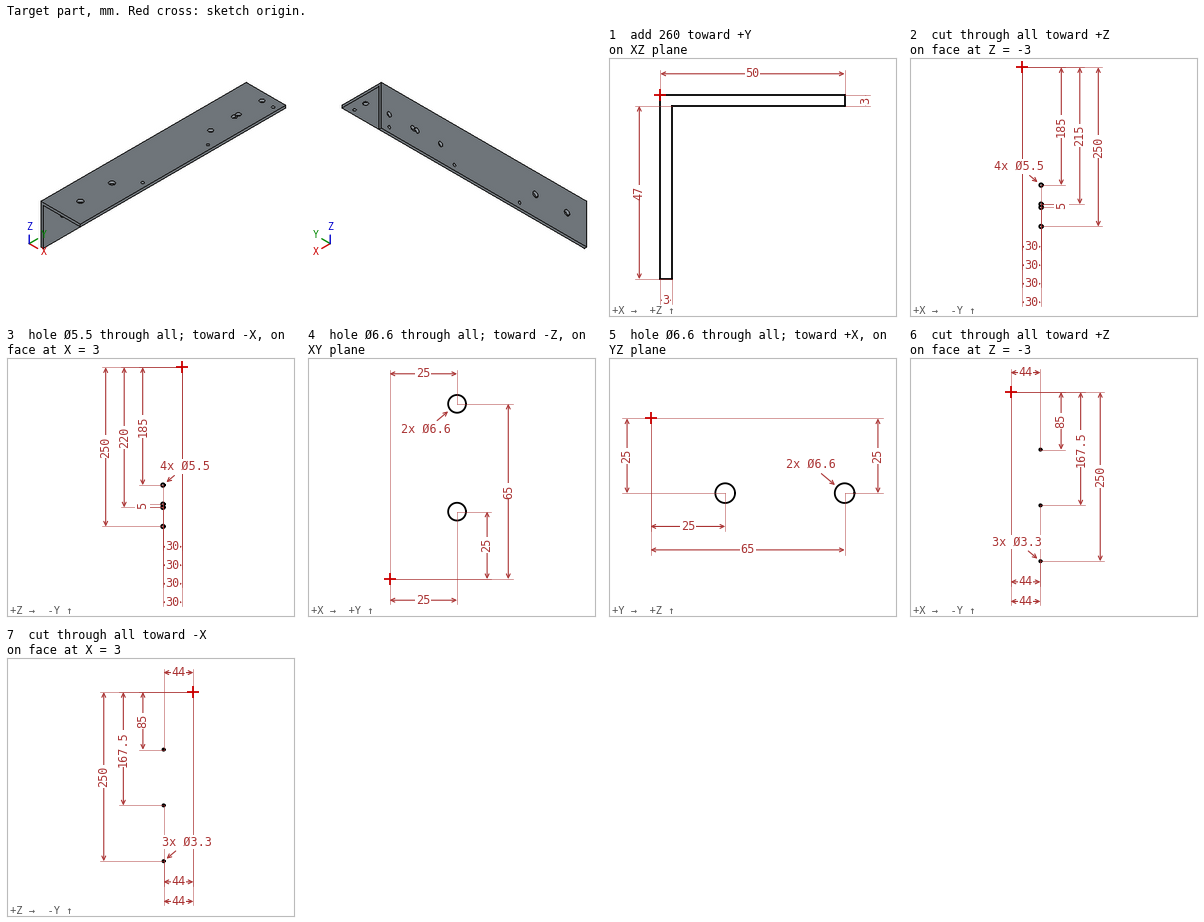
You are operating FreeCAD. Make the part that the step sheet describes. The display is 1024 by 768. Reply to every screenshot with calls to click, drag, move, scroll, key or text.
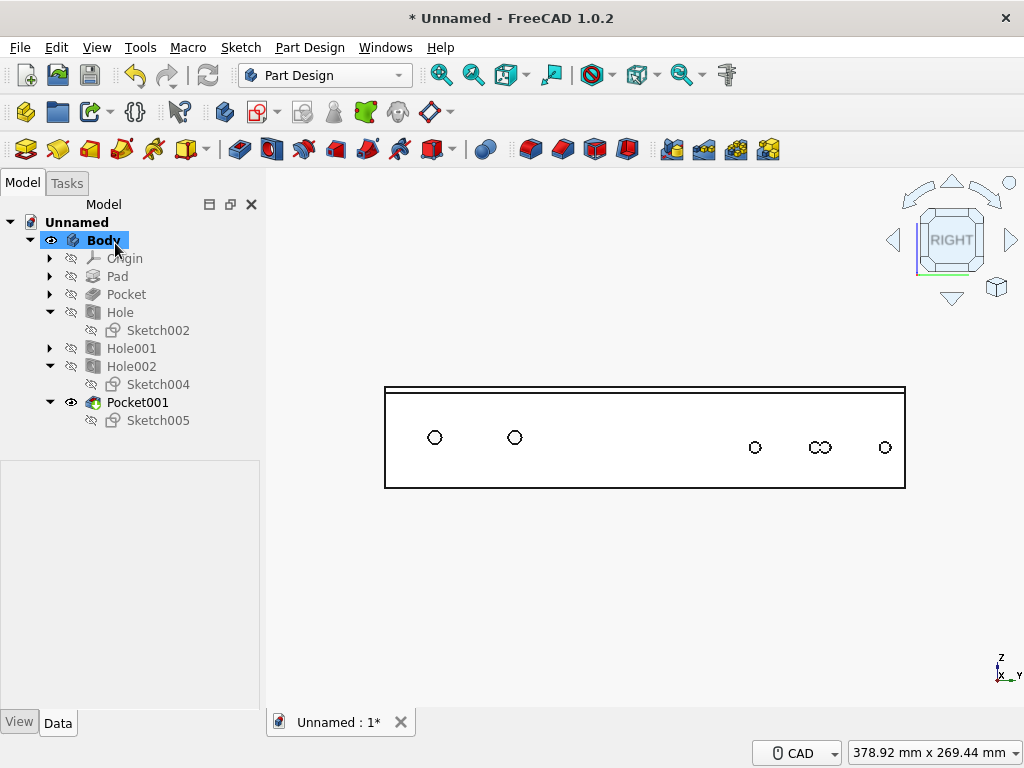
click(645, 440)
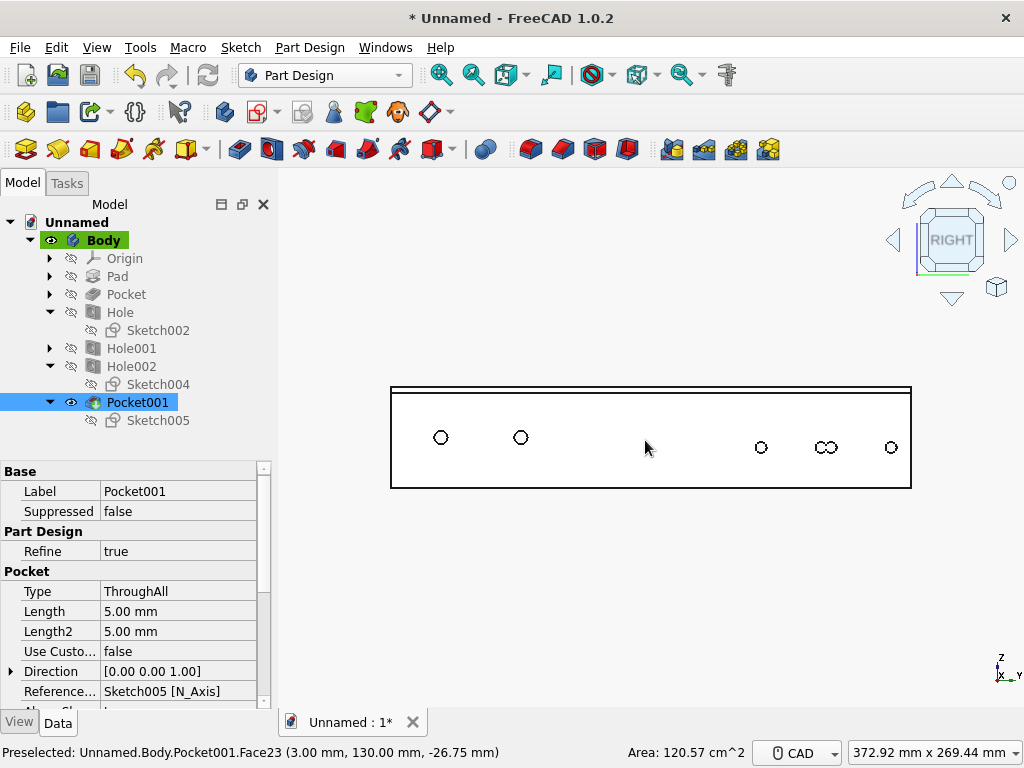
click(258, 112)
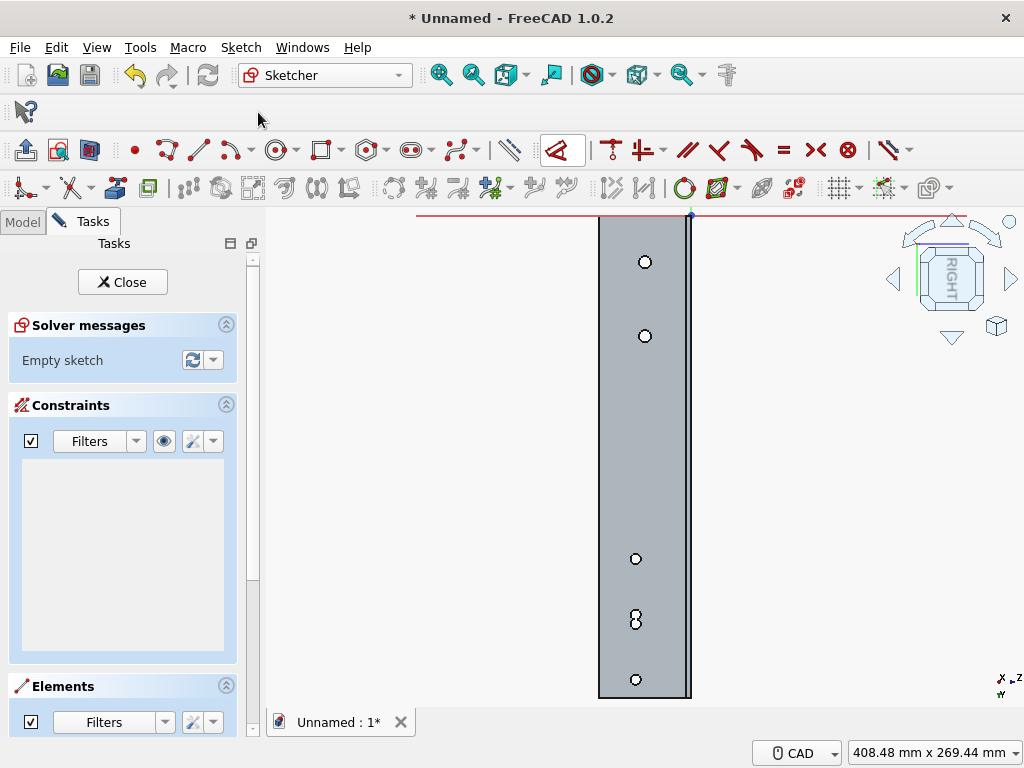
key(q)
key(s)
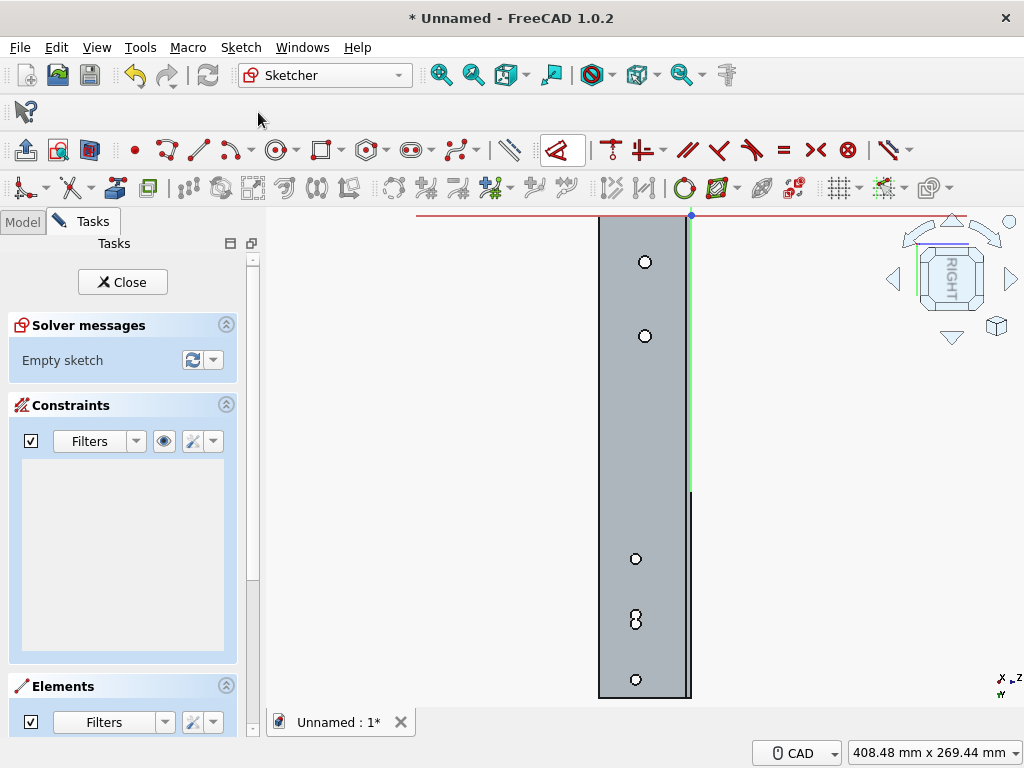
scroll(429, 473, down, 2)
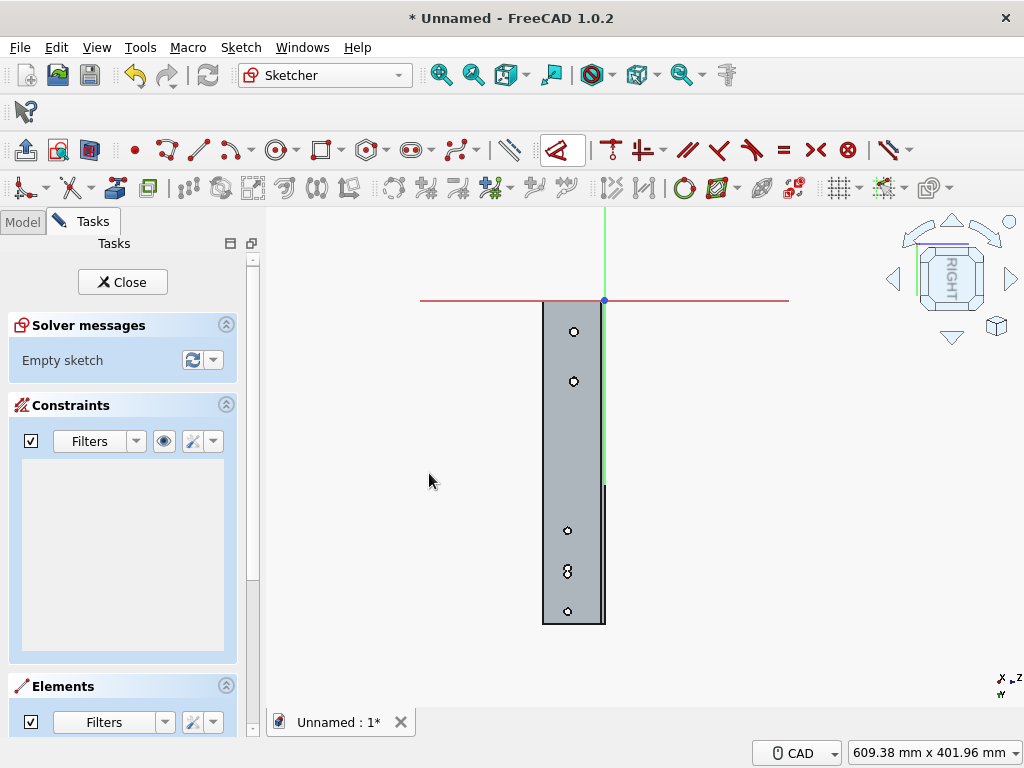
click(276, 150)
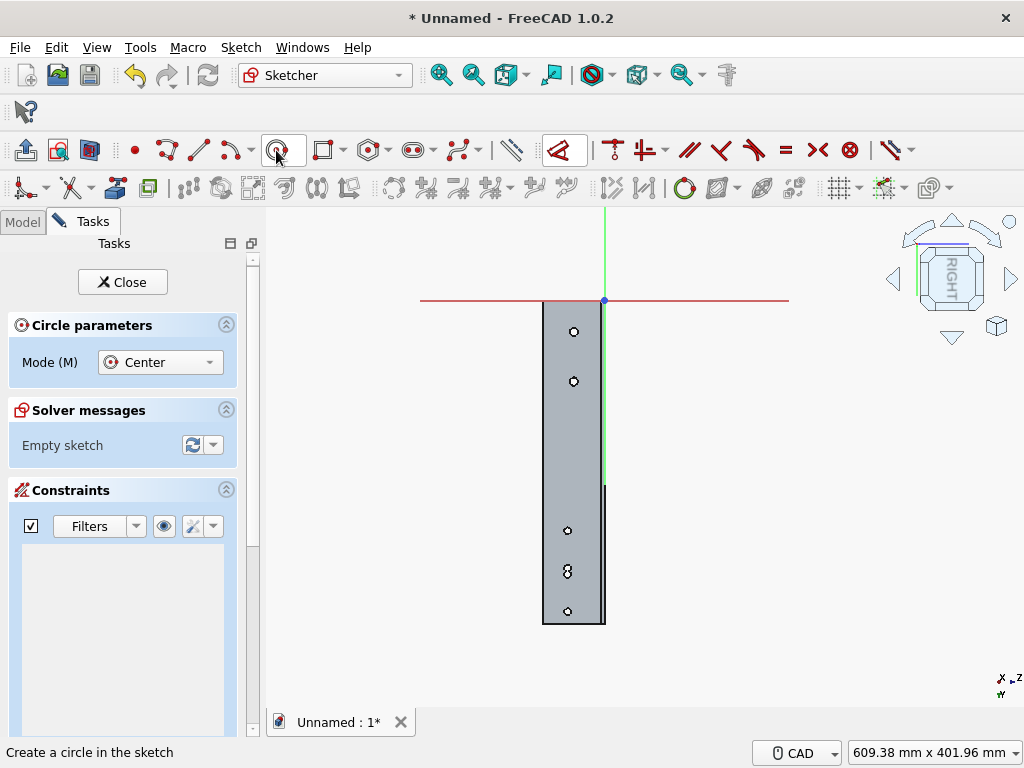
scroll(550, 612, up, 13)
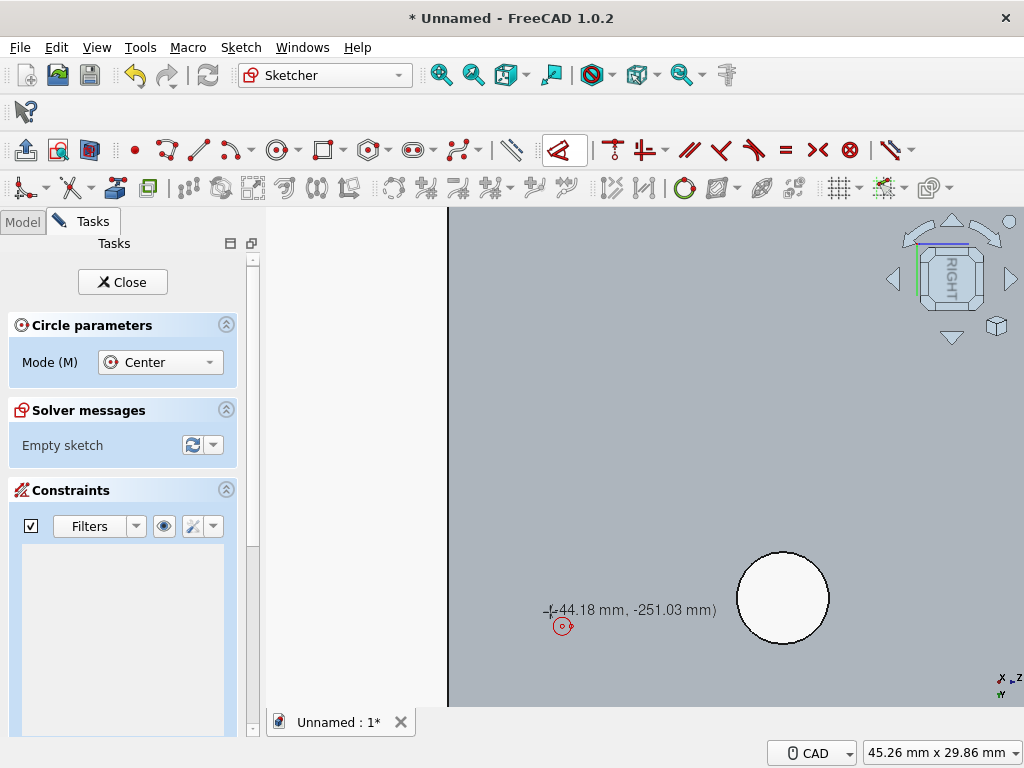
scroll(550, 613, down, 13)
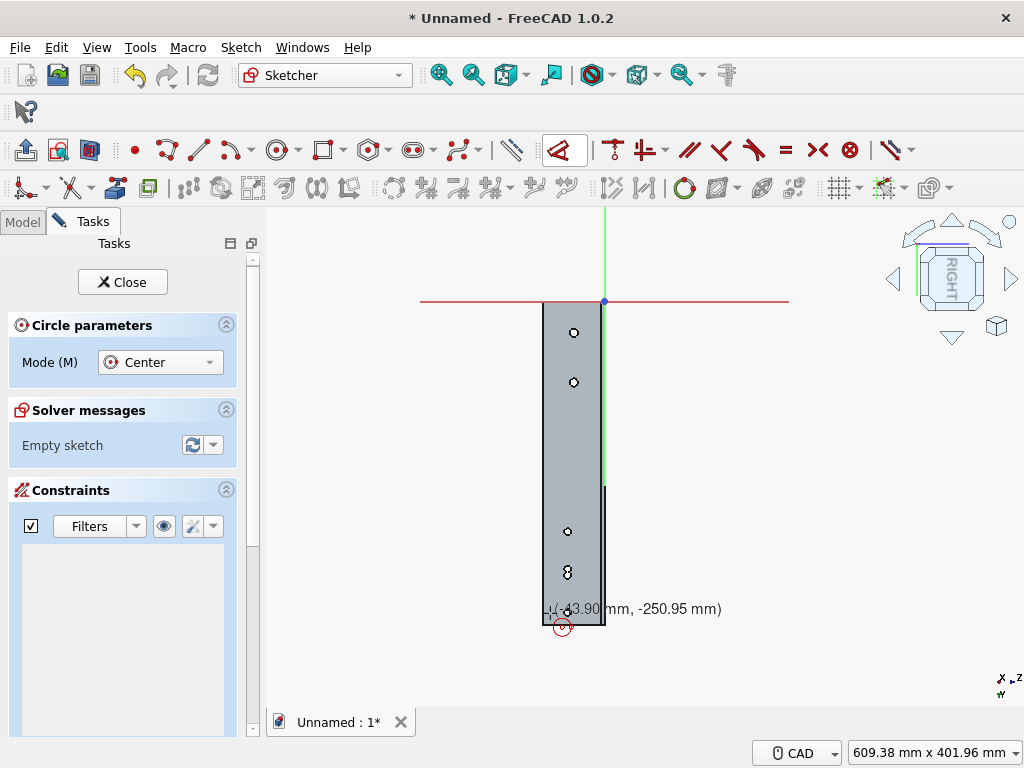
click(550, 613)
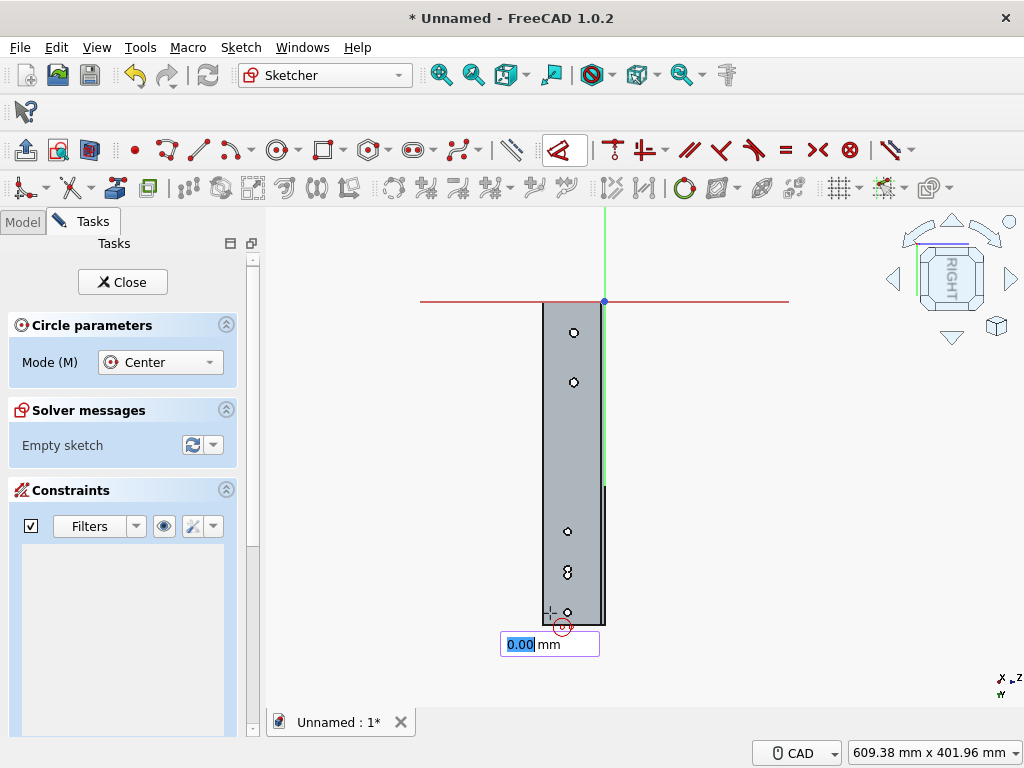
scroll(552, 611, up, 11)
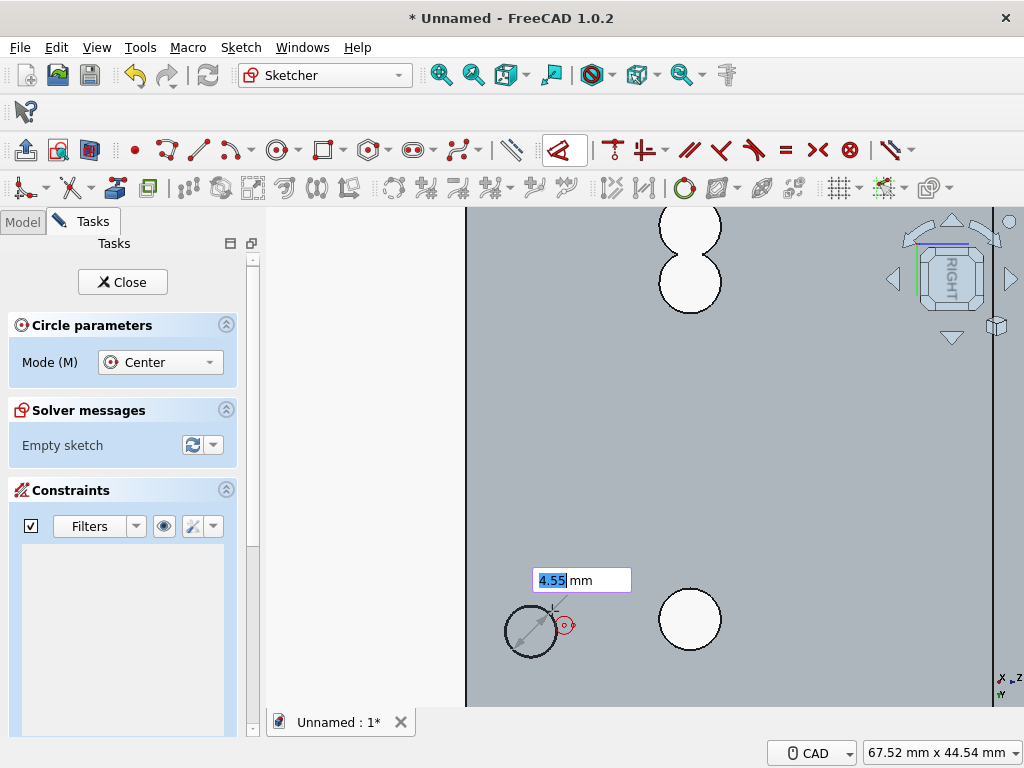
click(546, 606)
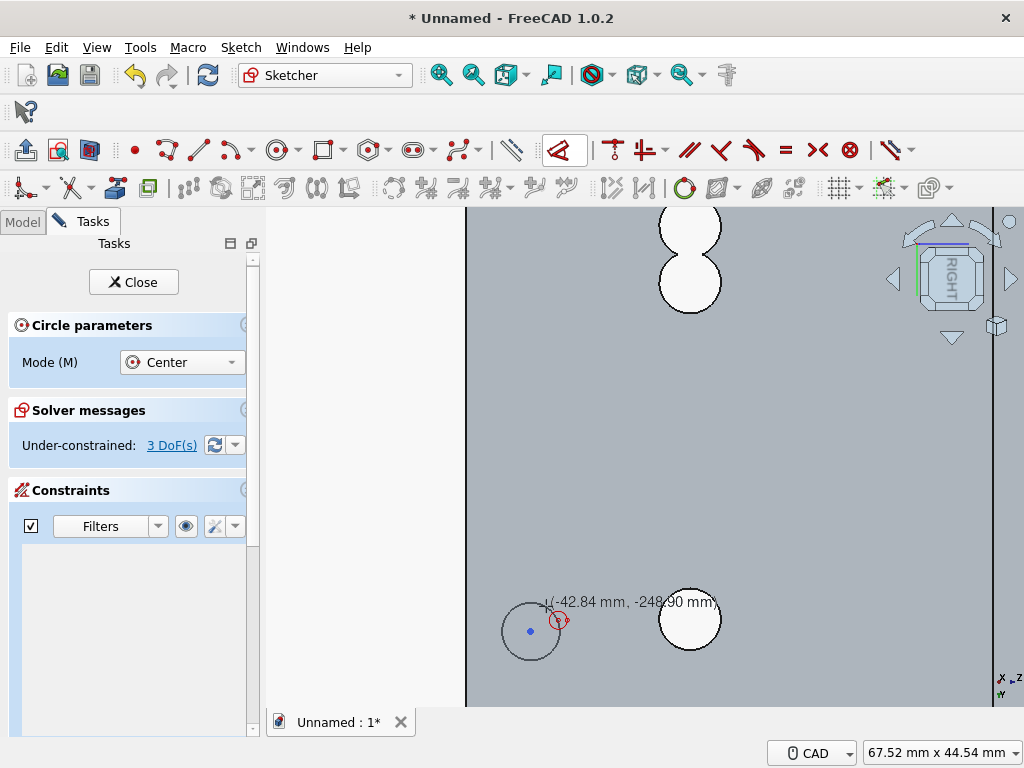
scroll(552, 610, down, 11)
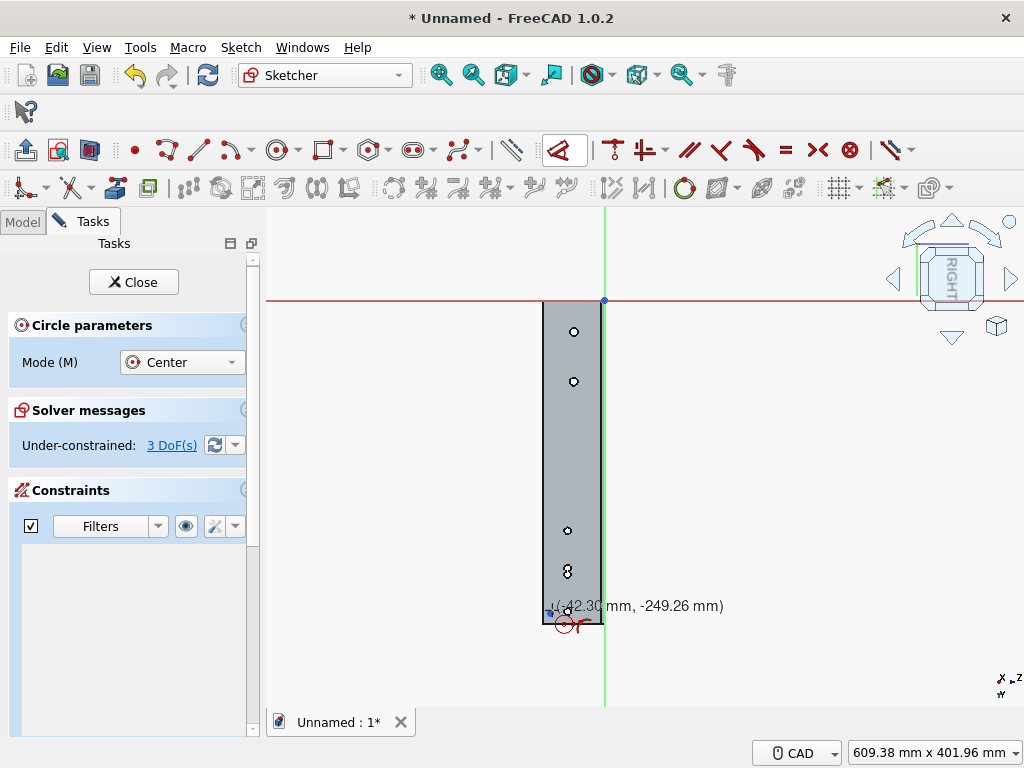
scroll(550, 509, up, 13)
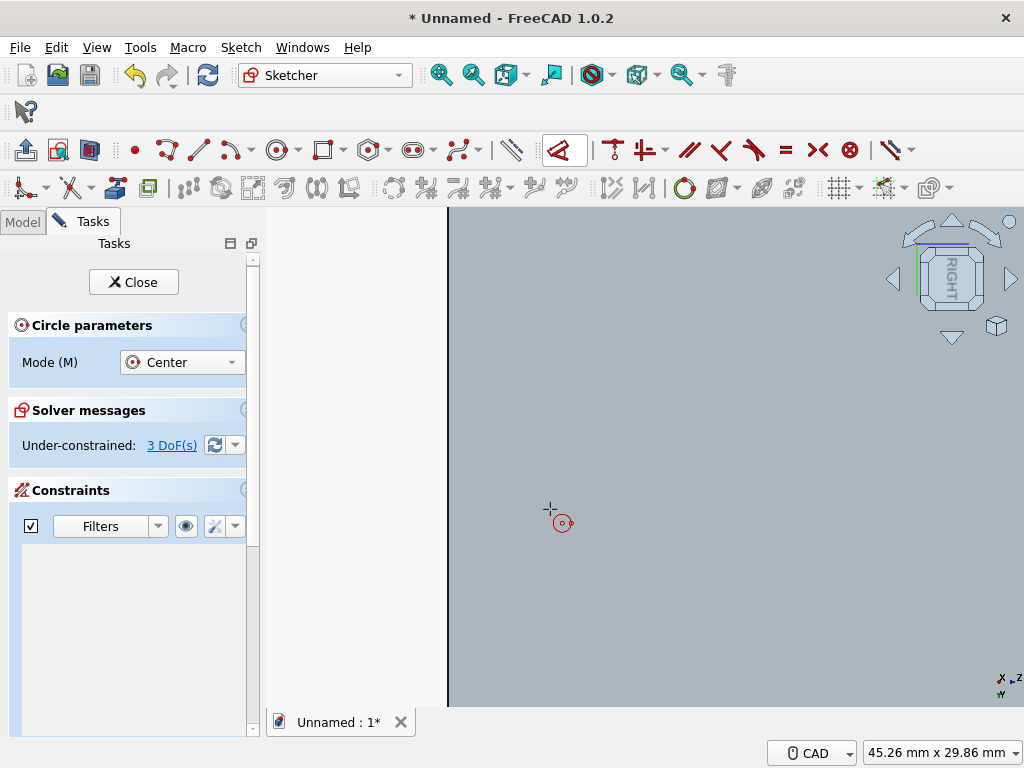
scroll(550, 509, down, 13)